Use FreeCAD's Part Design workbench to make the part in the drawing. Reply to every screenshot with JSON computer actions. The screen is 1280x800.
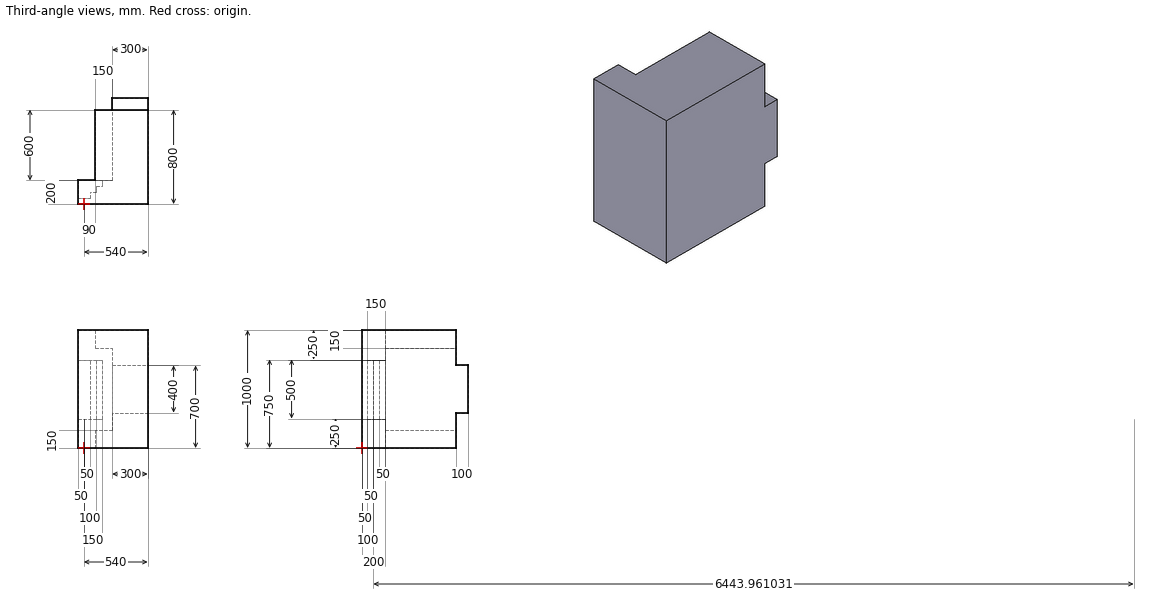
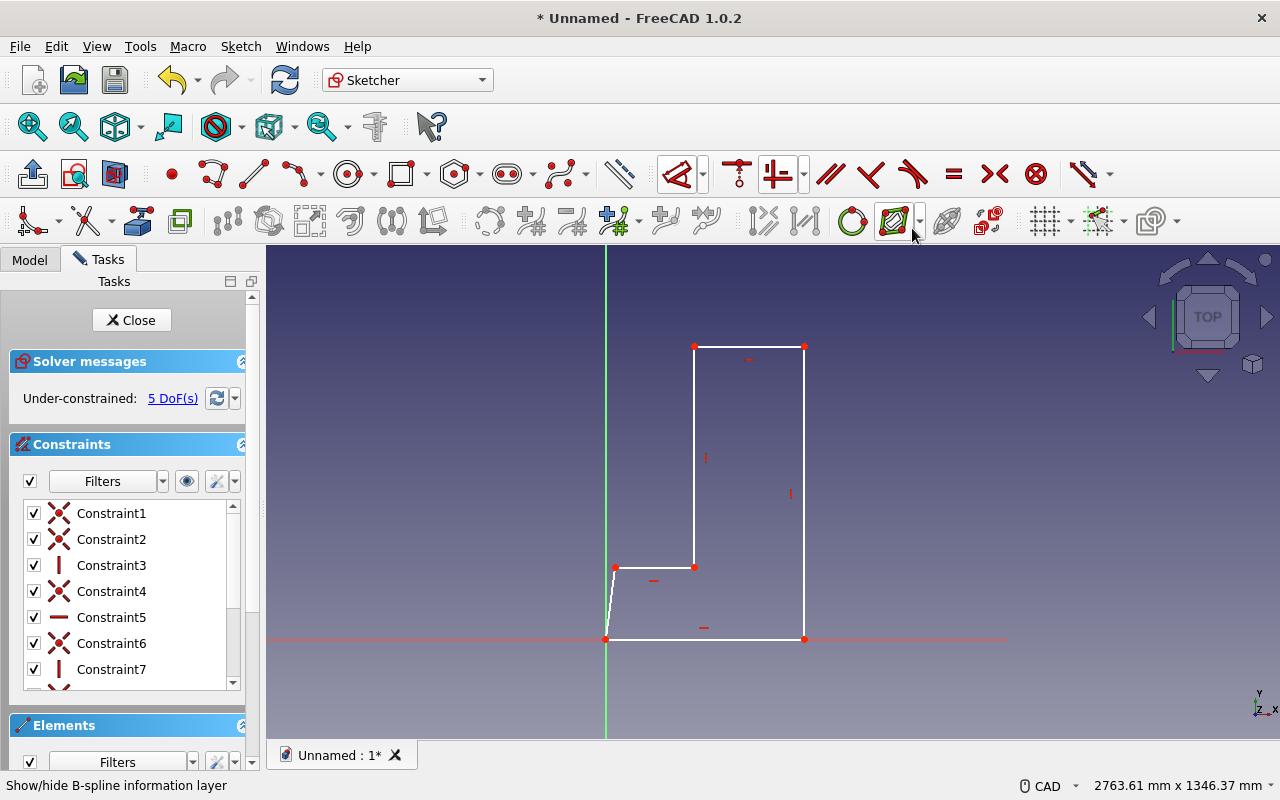
{"action": "left_click", "coordinate": [609, 618]}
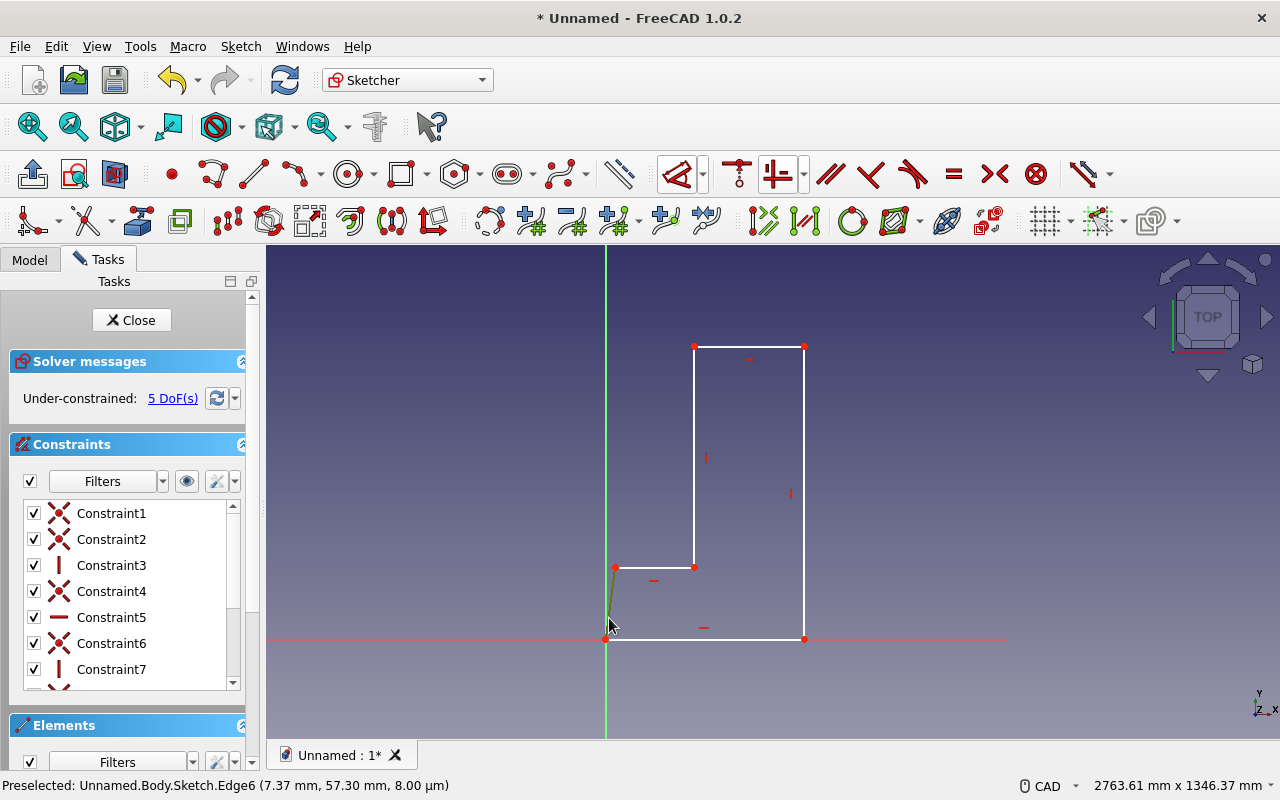
{"action": "left_click", "coordinate": [804, 174]}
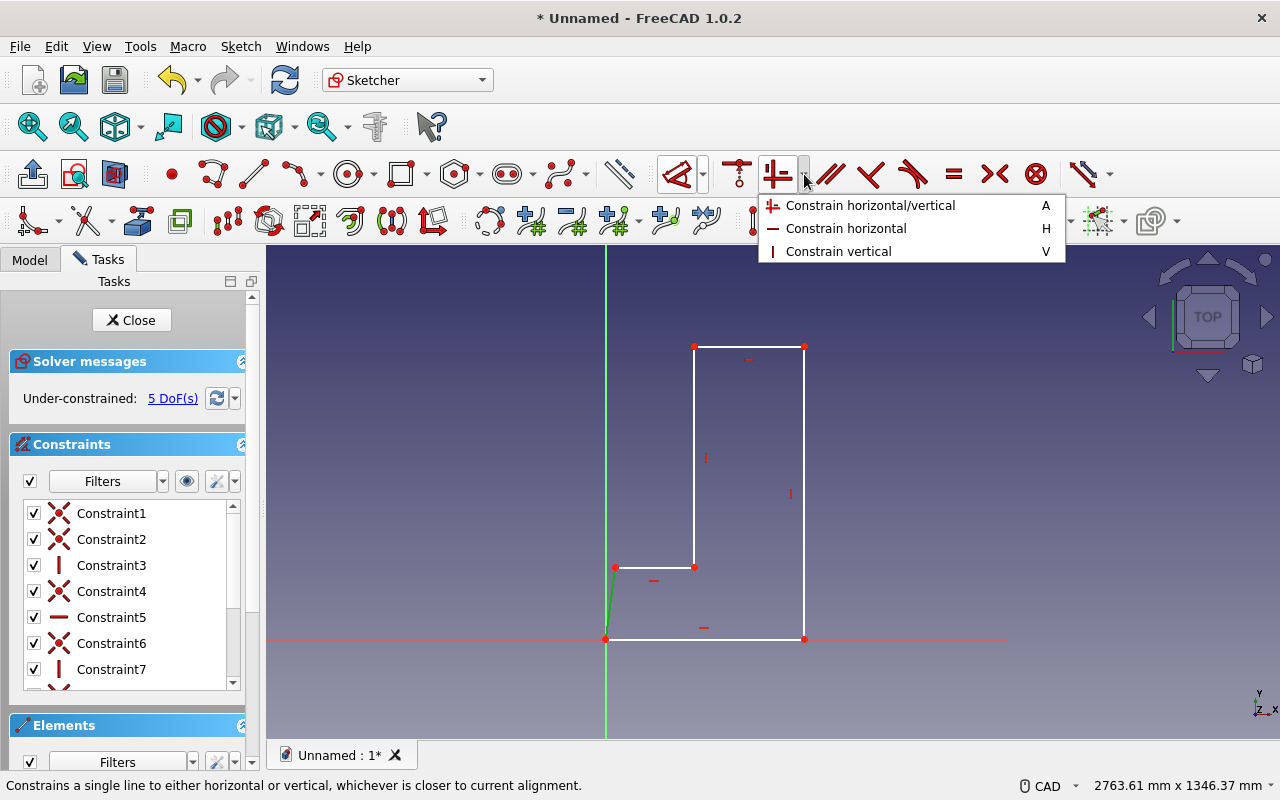
{"action": "left_click", "coordinate": [912, 252]}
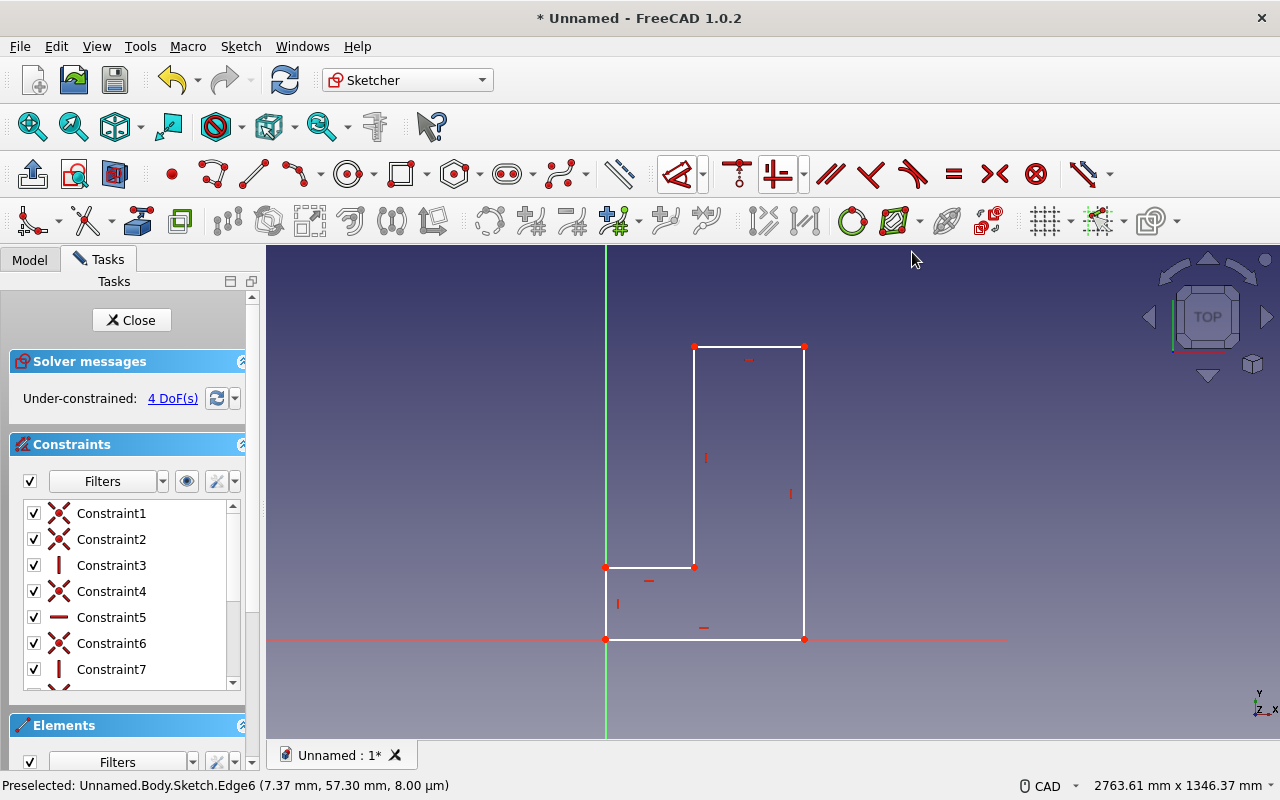
{"action": "left_click", "coordinate": [665, 640]}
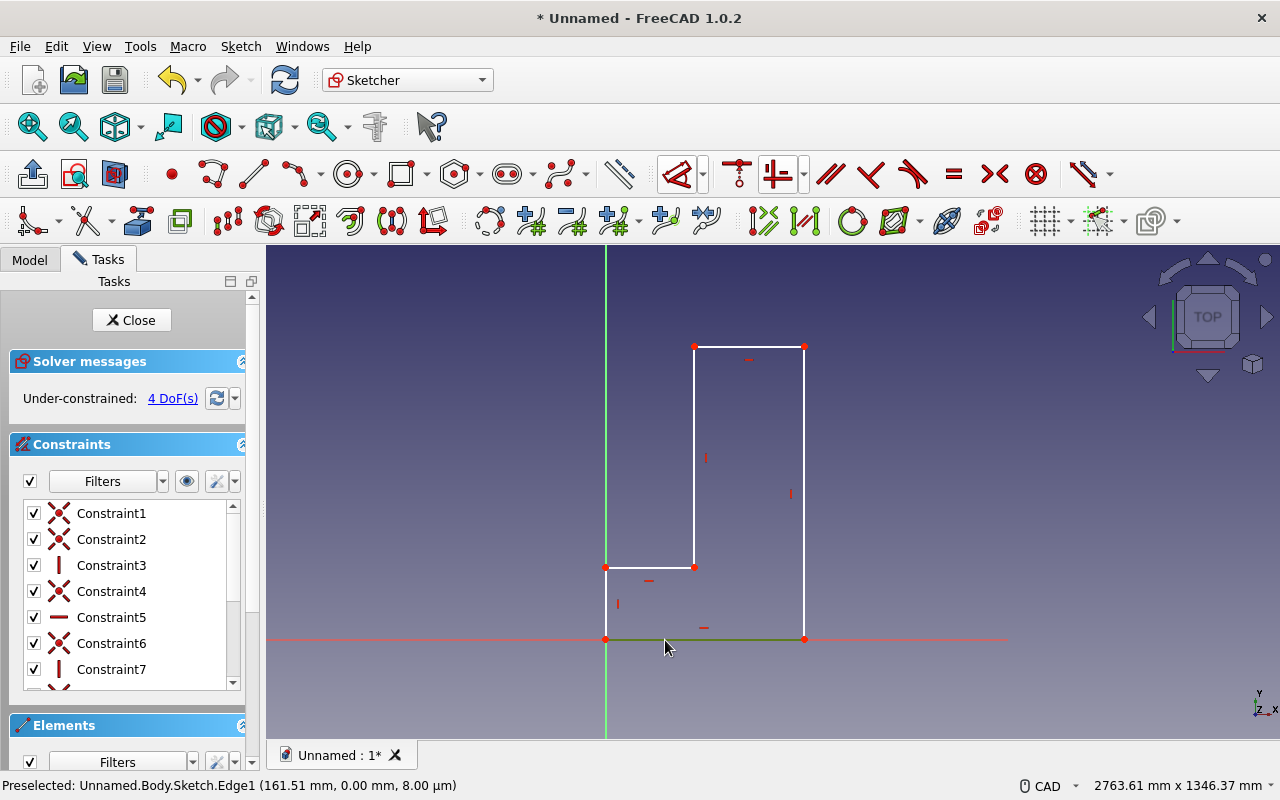
{"action": "left_click", "coordinate": [702, 174]}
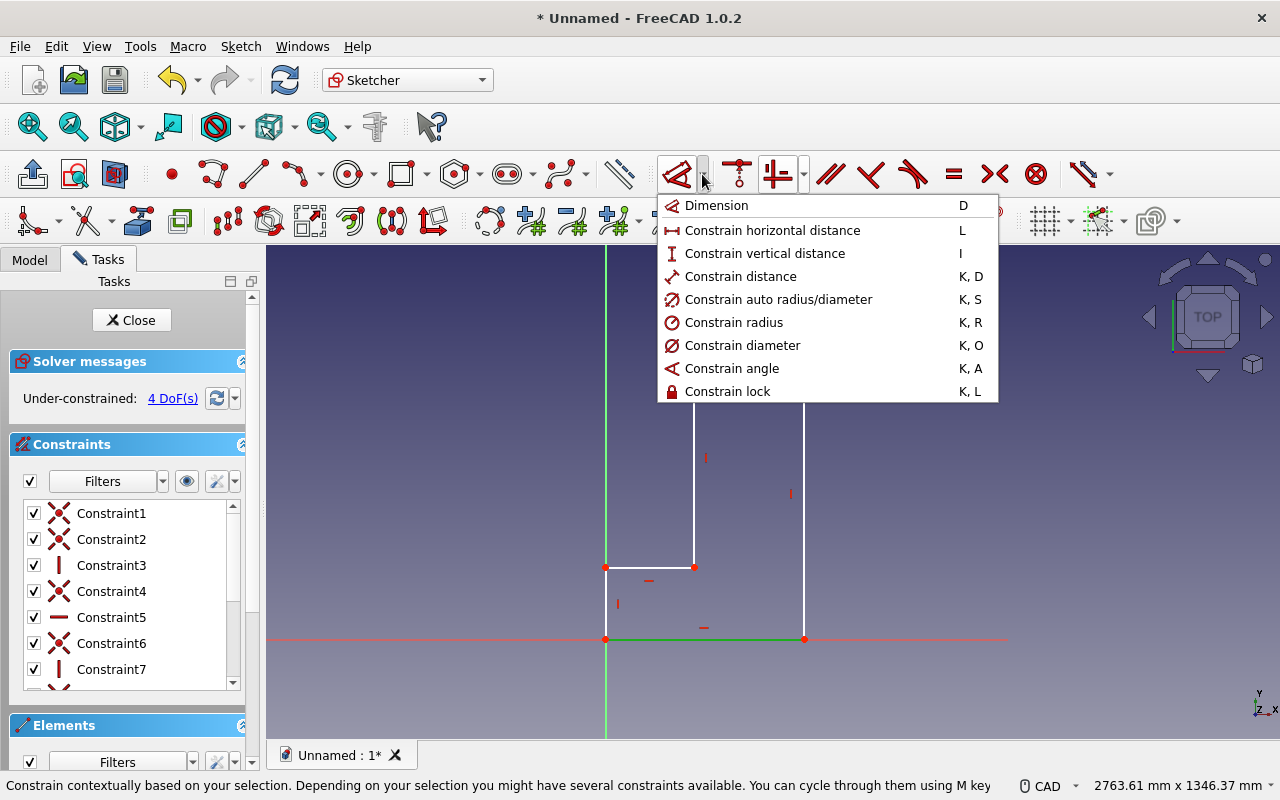
{"action": "left_click", "coordinate": [828, 230]}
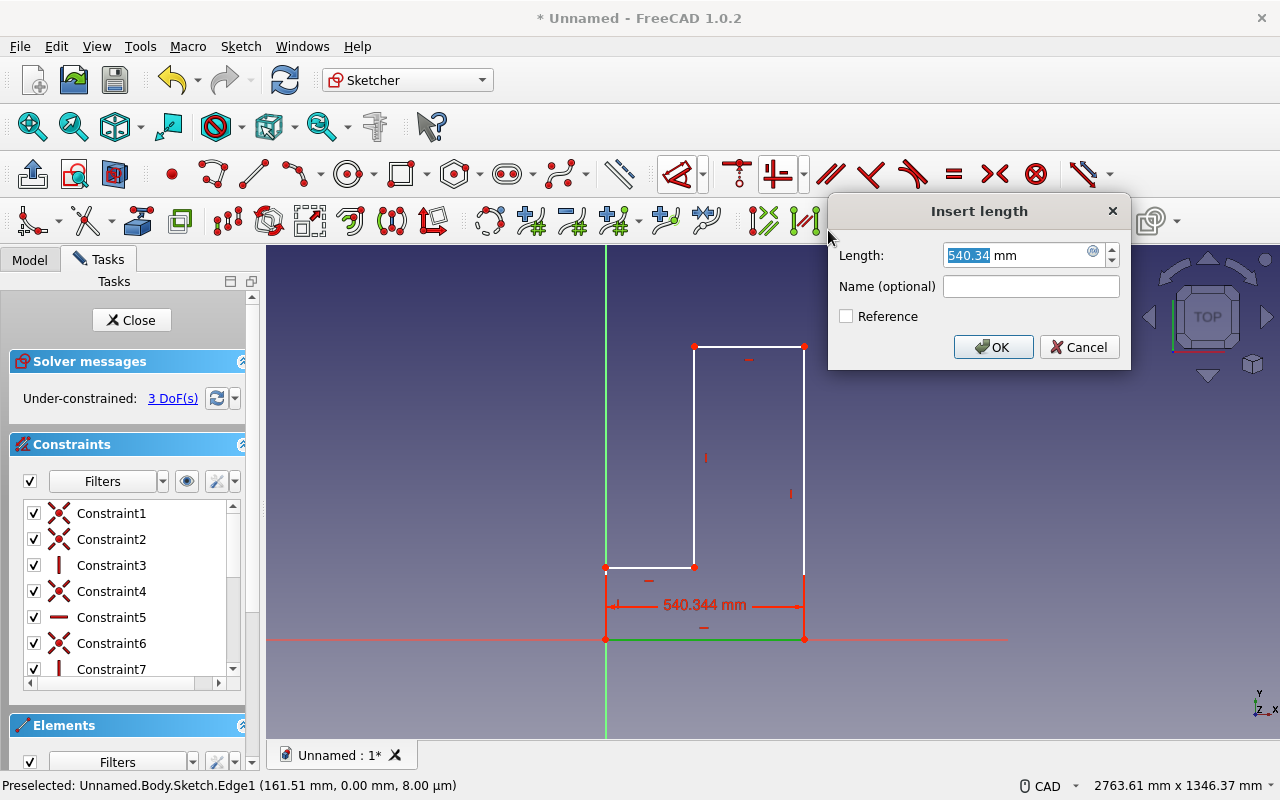
{"action": "type", "text": "540"}
{"action": "key", "text": "Return"}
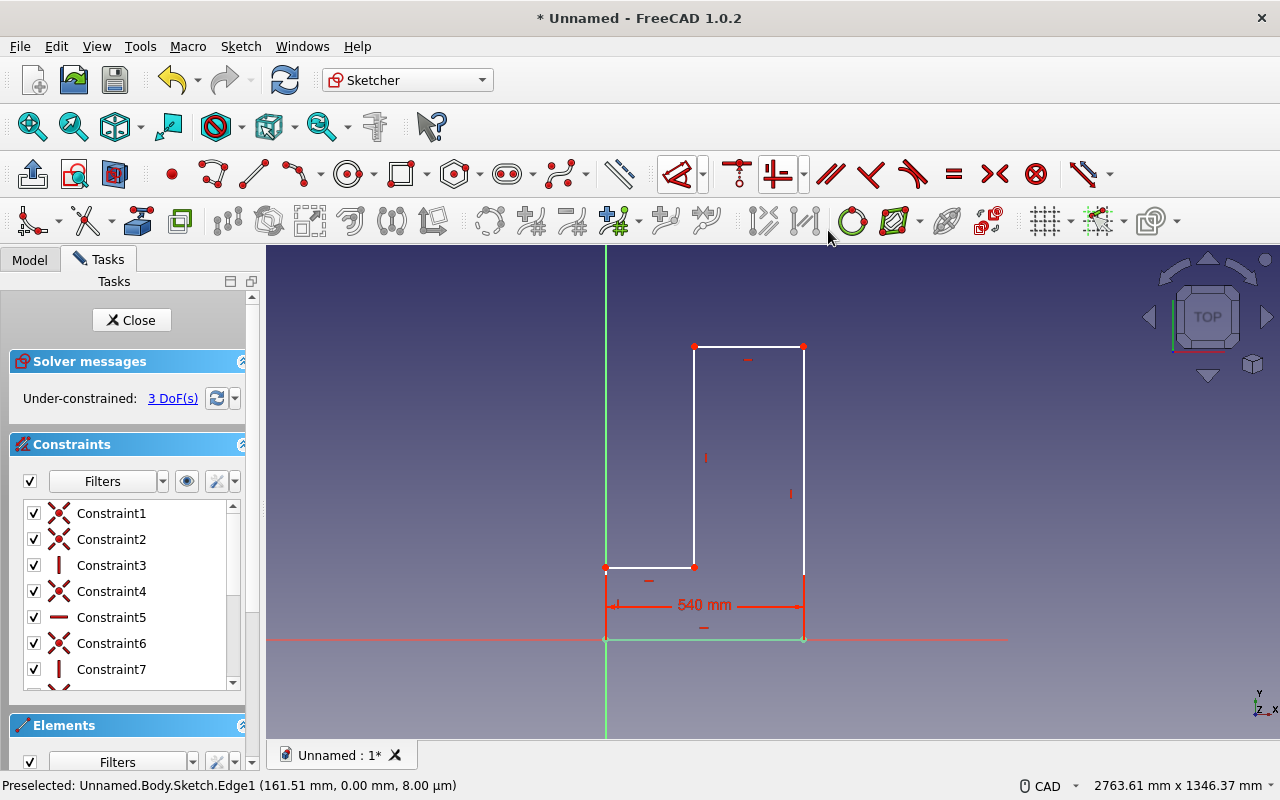
{"action": "left_click", "coordinate": [804, 552]}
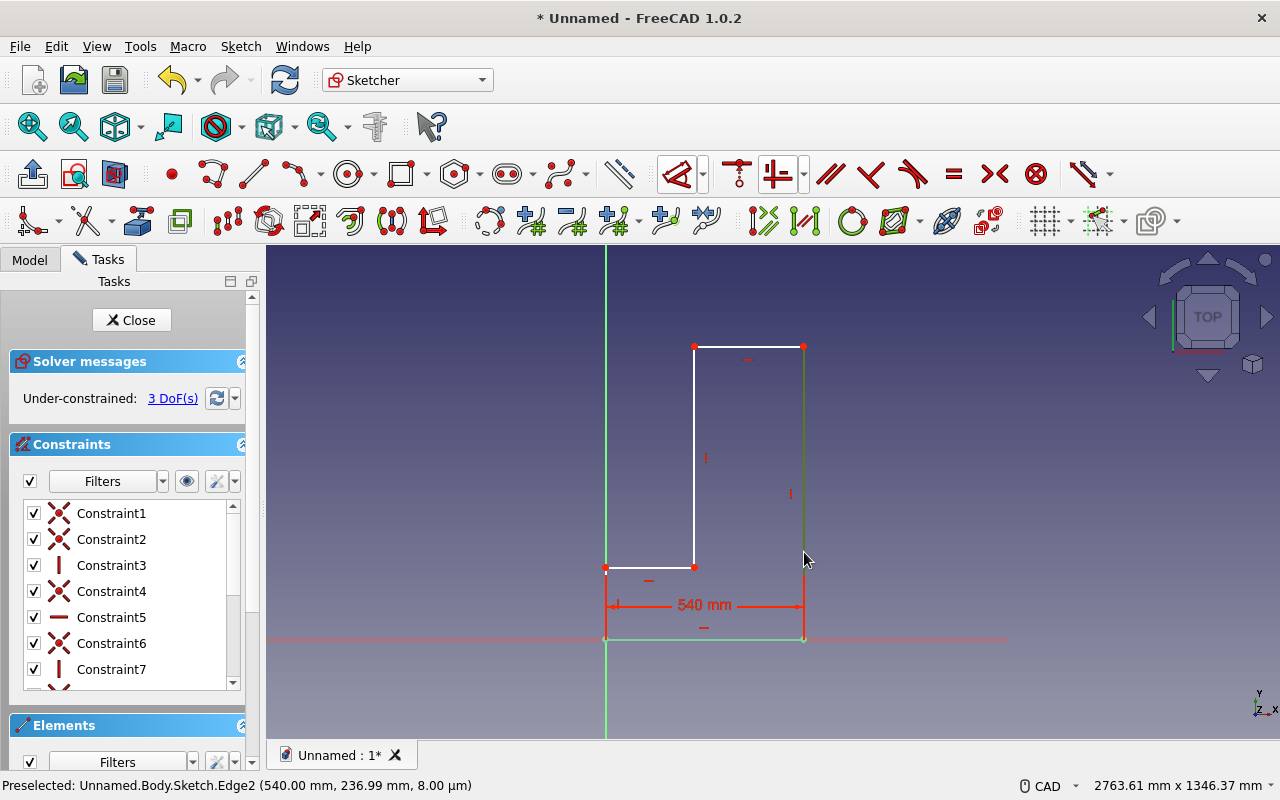
{"action": "left_click", "coordinate": [702, 174]}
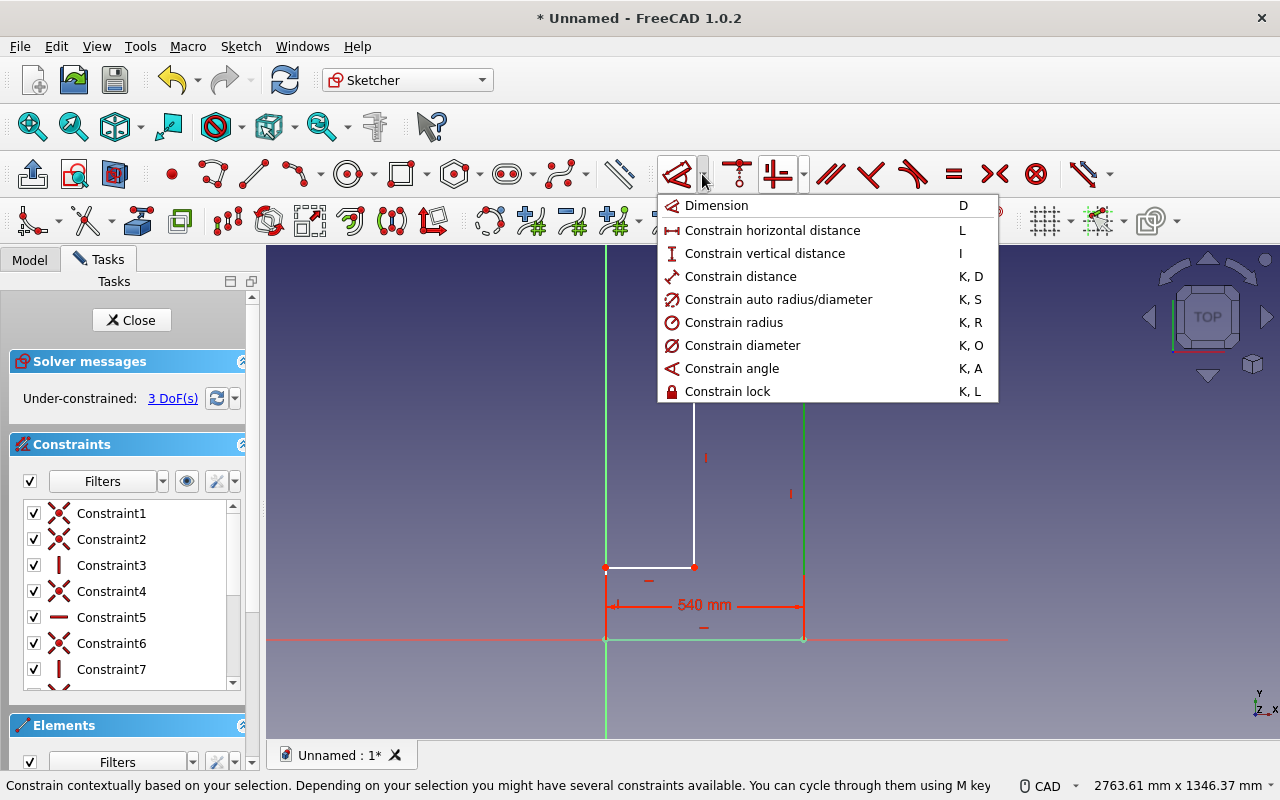
{"action": "left_click", "coordinate": [828, 254]}